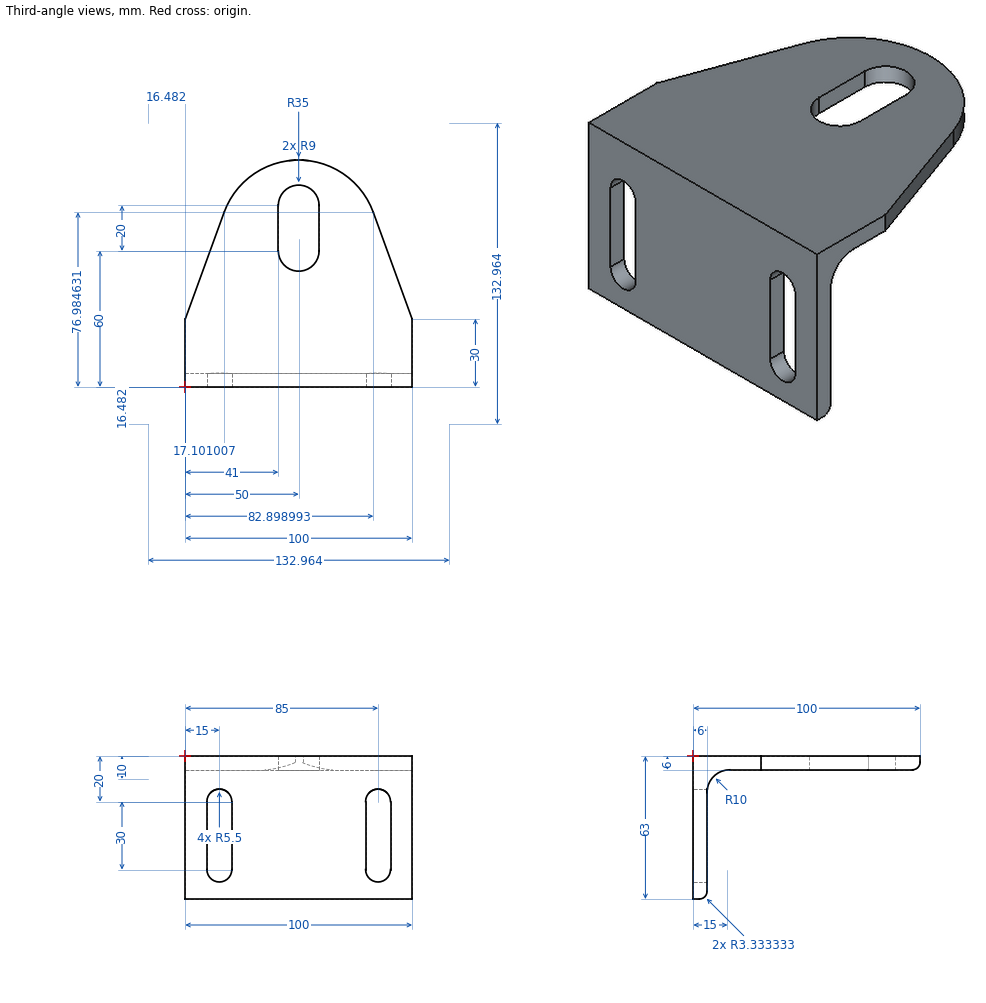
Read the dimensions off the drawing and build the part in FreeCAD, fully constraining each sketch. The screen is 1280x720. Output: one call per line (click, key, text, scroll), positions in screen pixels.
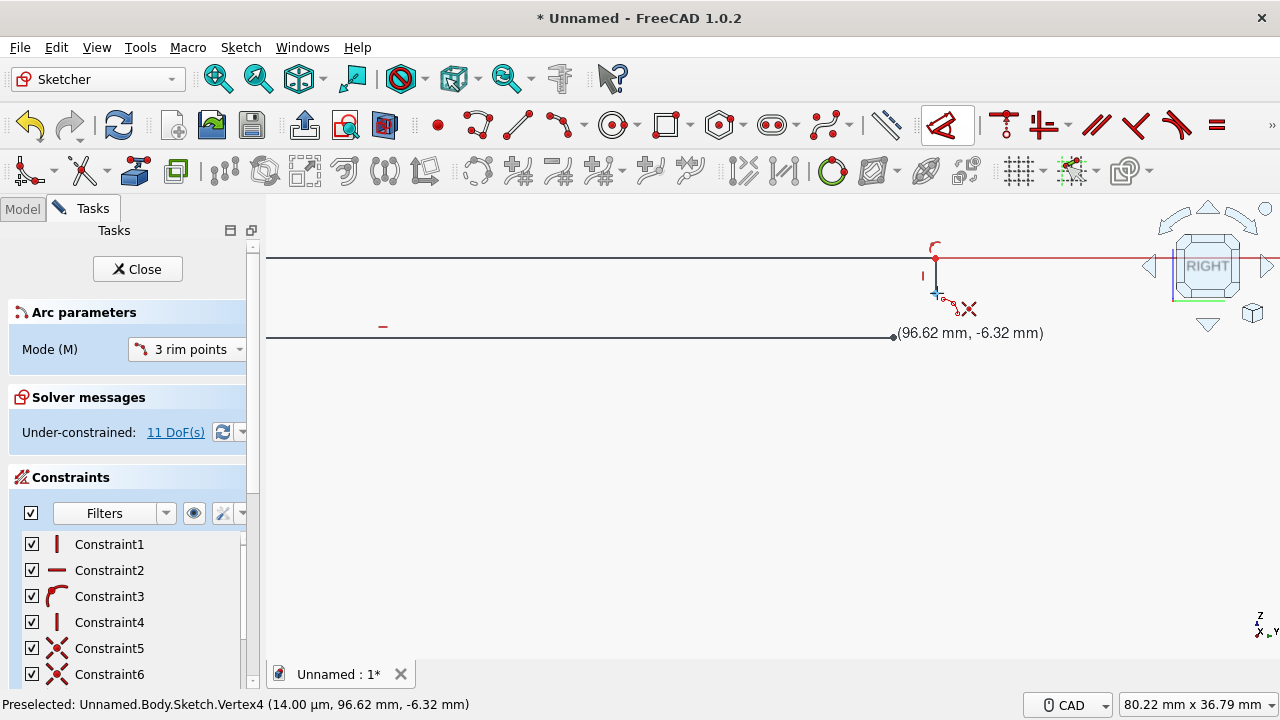
click(936, 294)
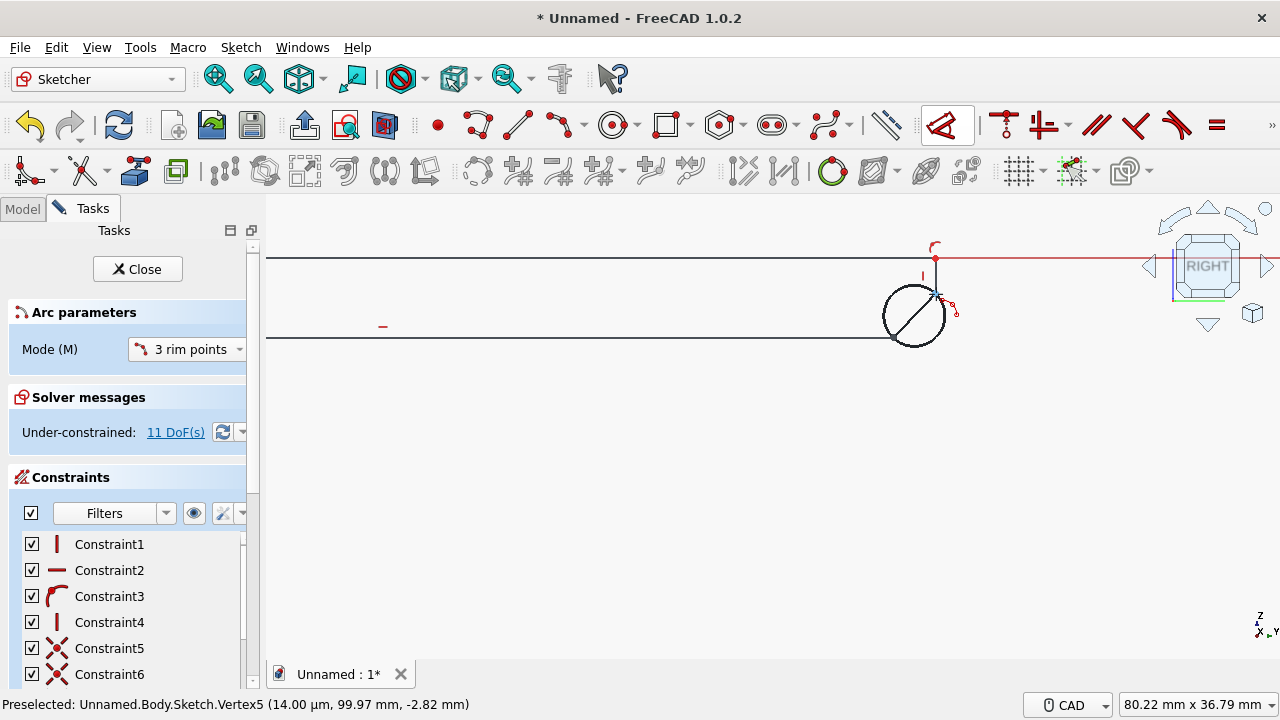
scroll(924, 322, up, 2)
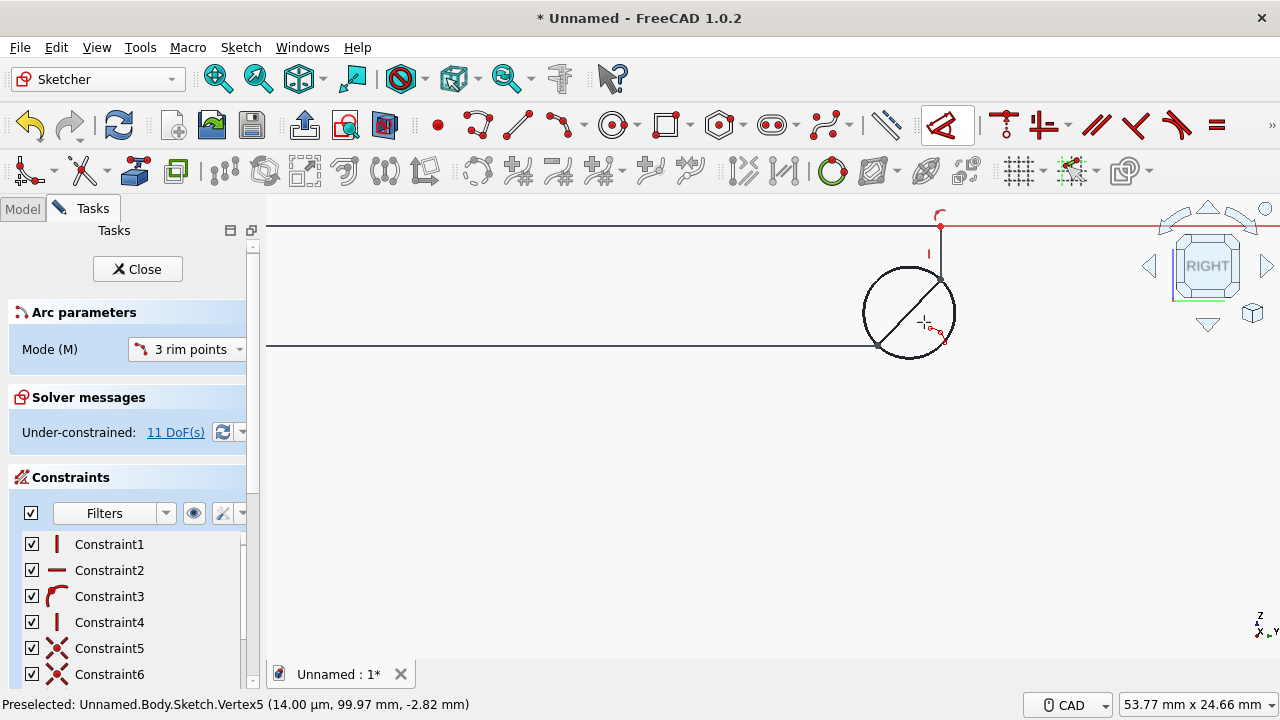
click(923, 321)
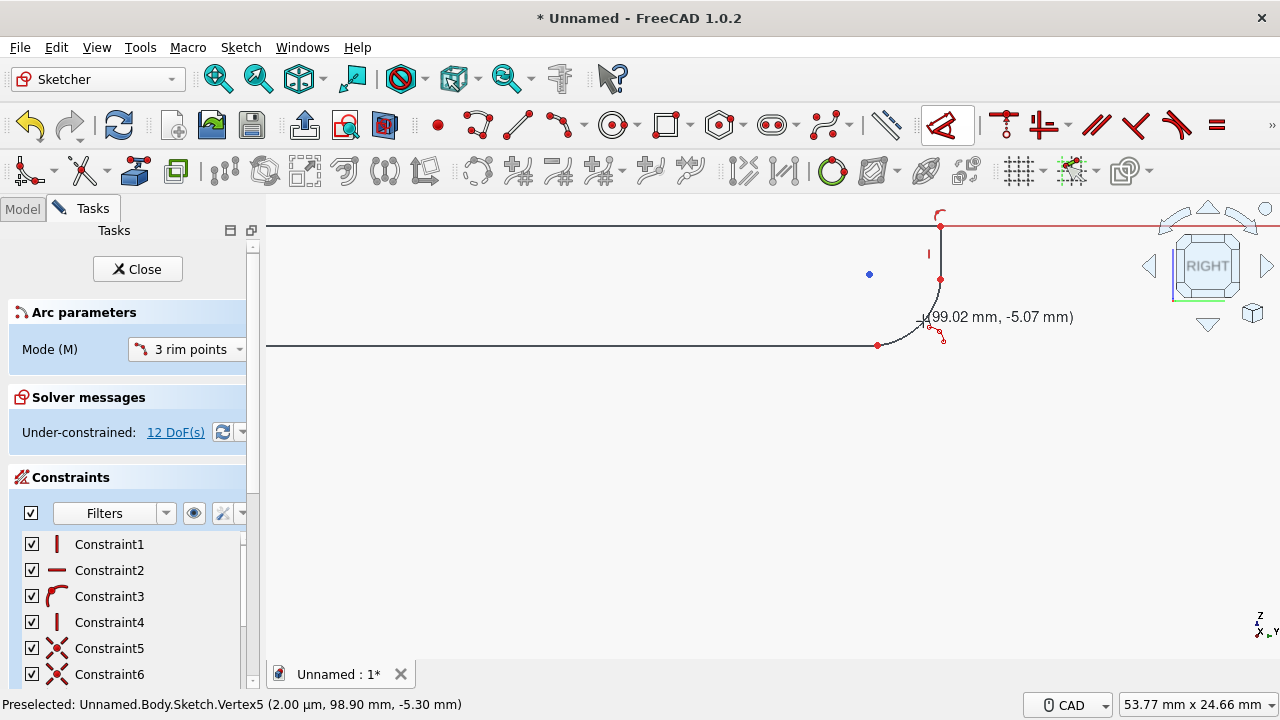
scroll(936, 298, down, 7)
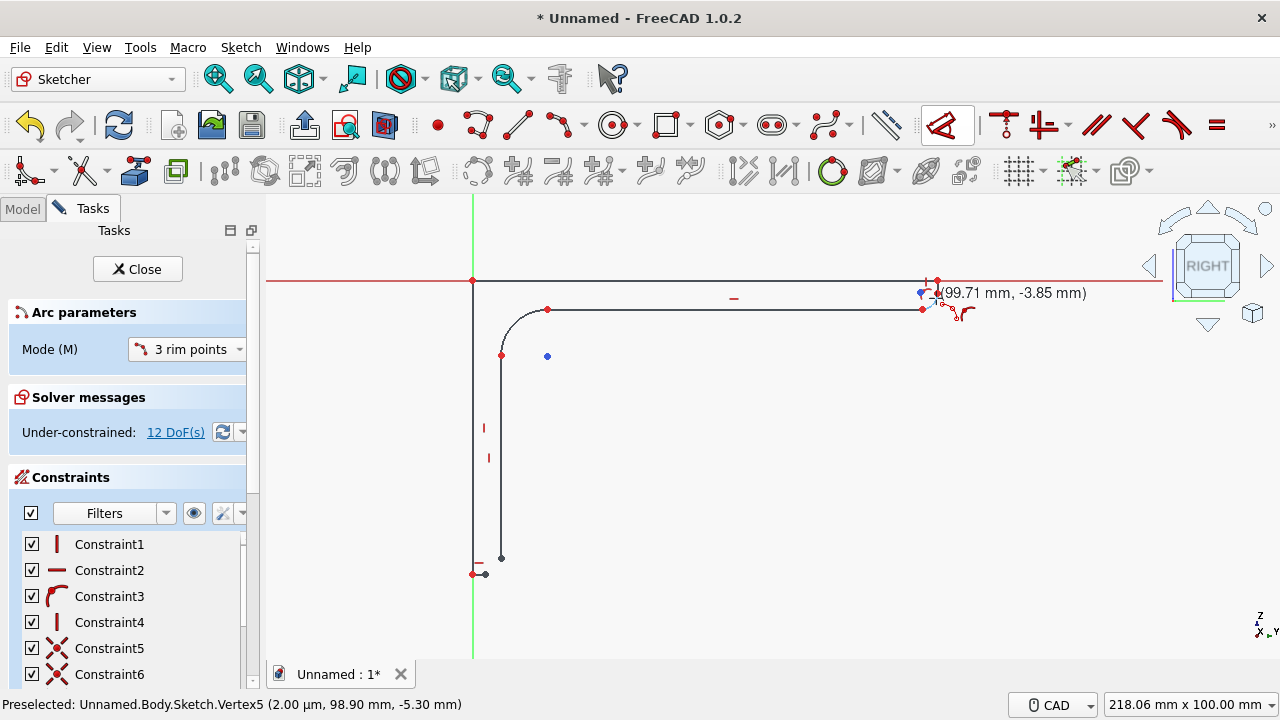
scroll(485, 573, up, 5)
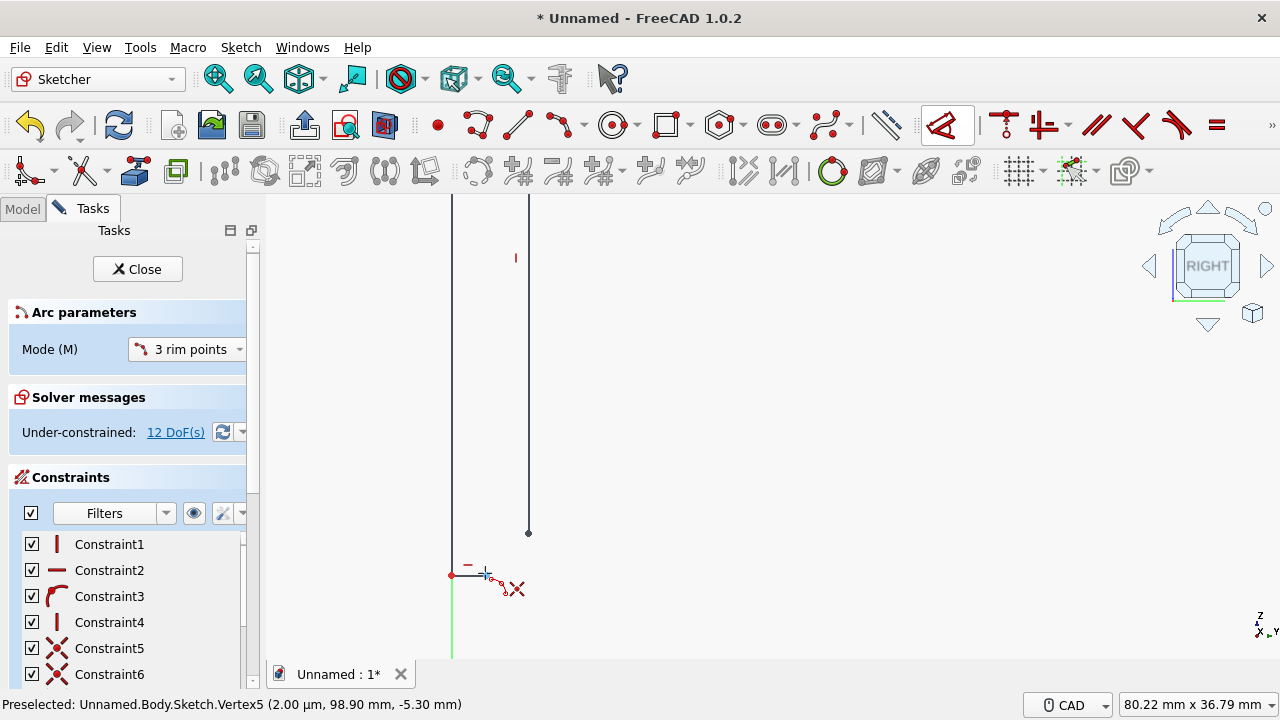
click(486, 576)
click(529, 533)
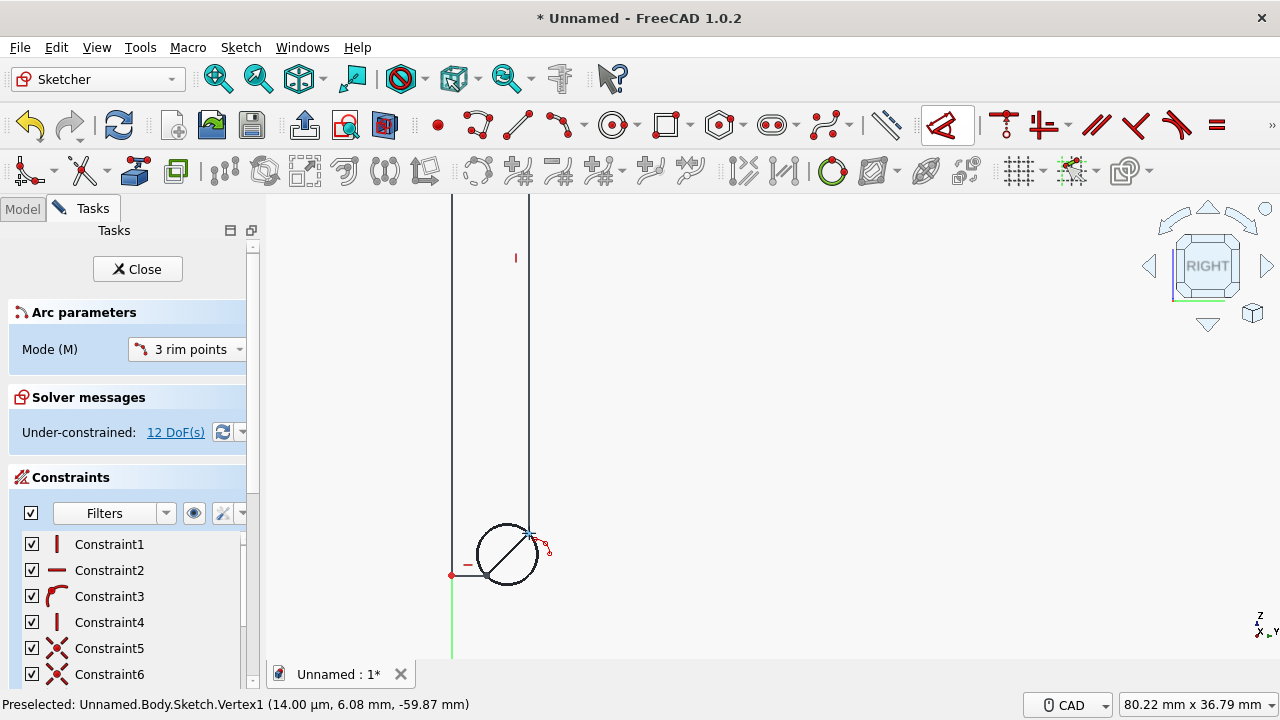
scroll(515, 561, up, 2)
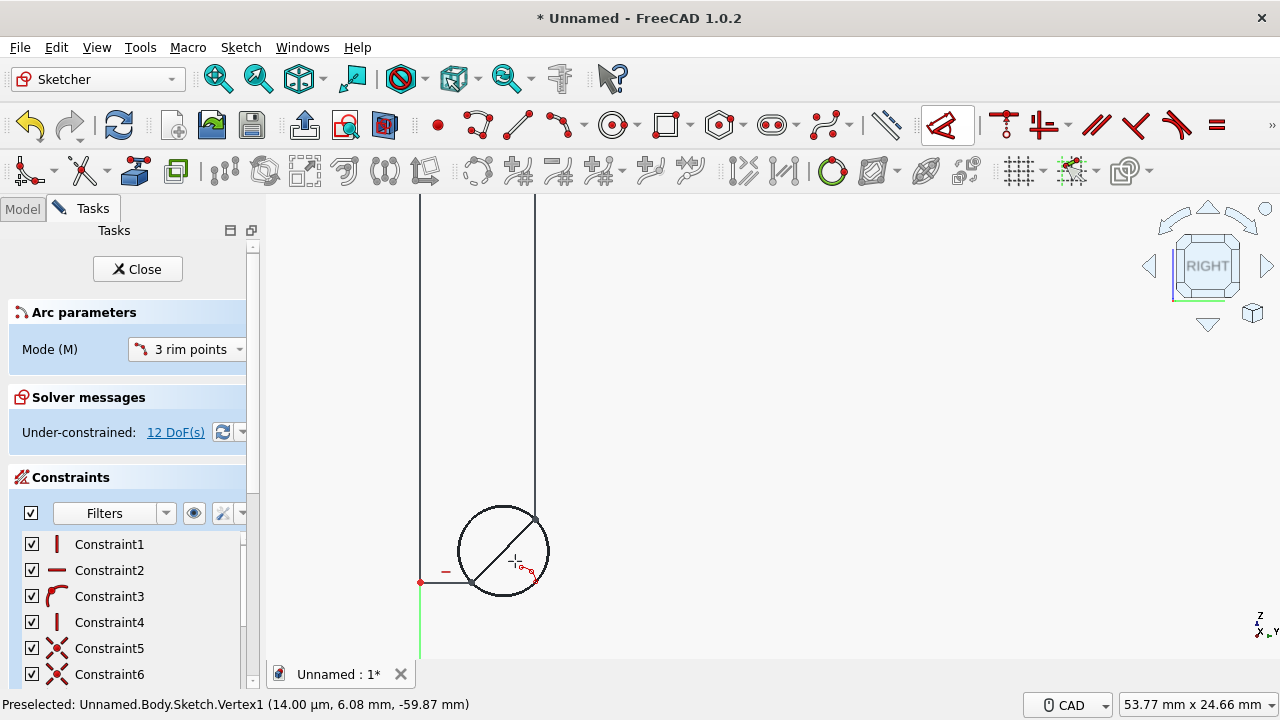
click(515, 560)
key(Escape)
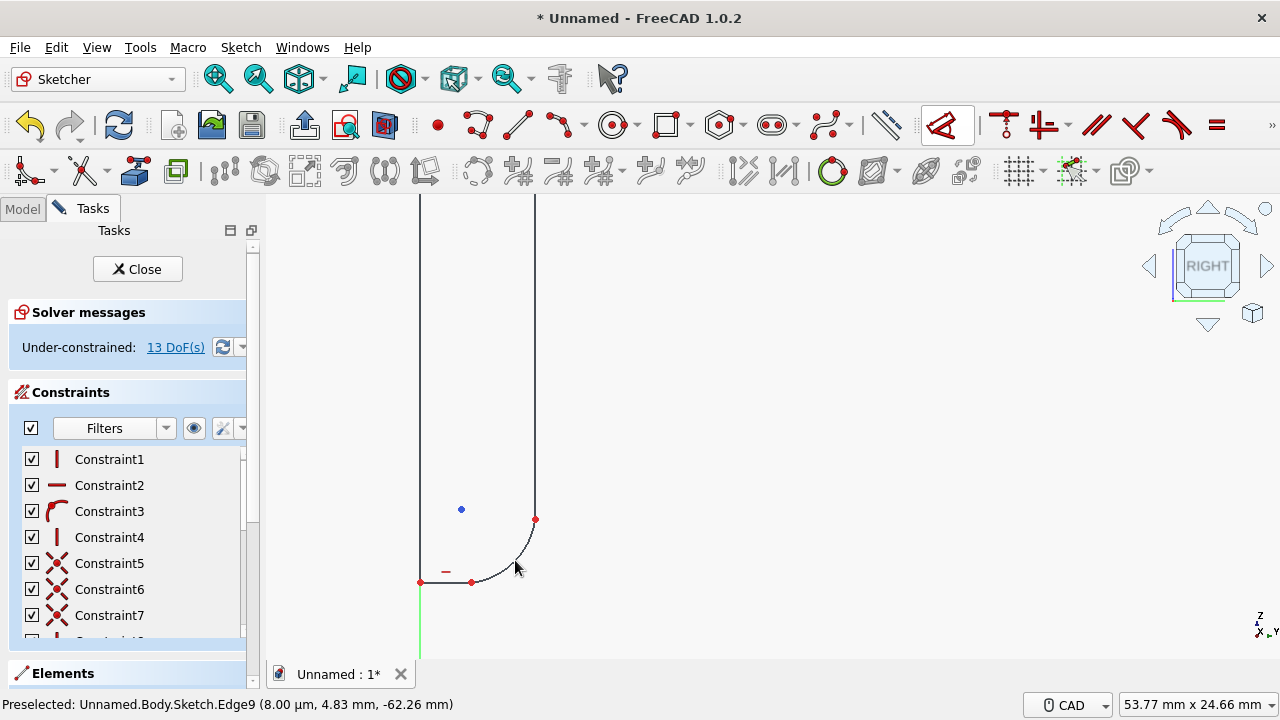
scroll(489, 571, down, 7)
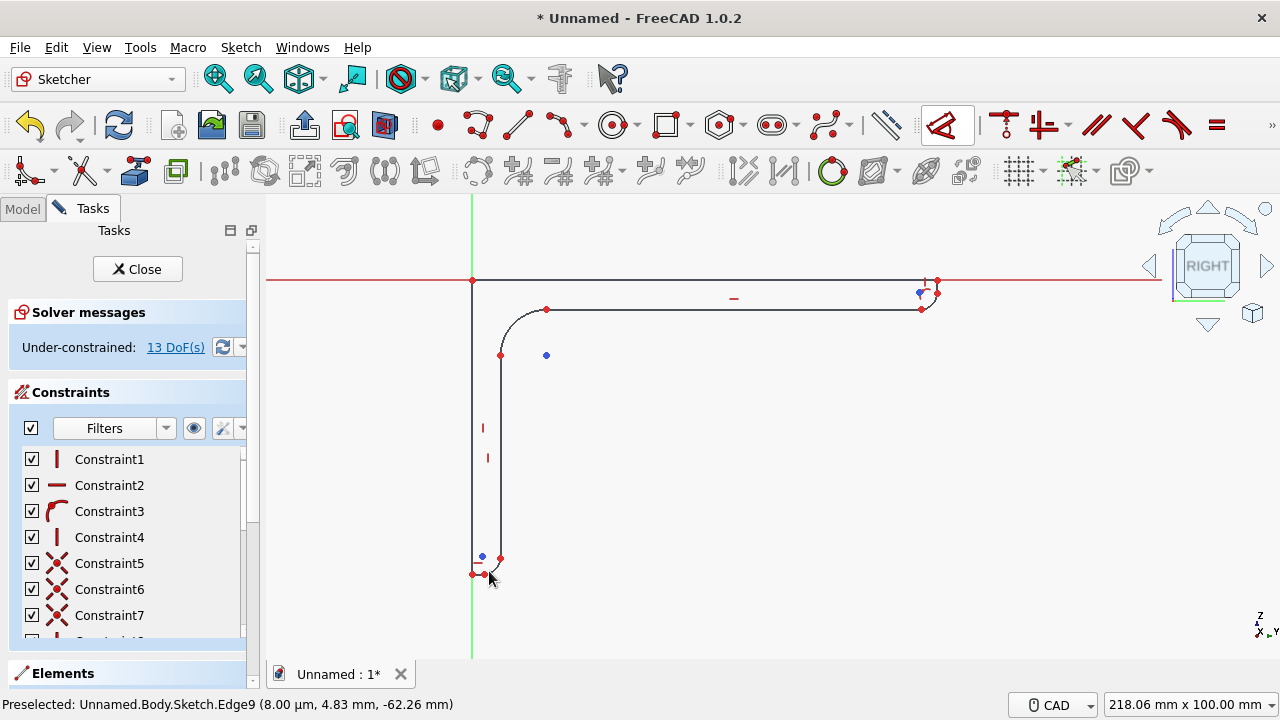
click(501, 498)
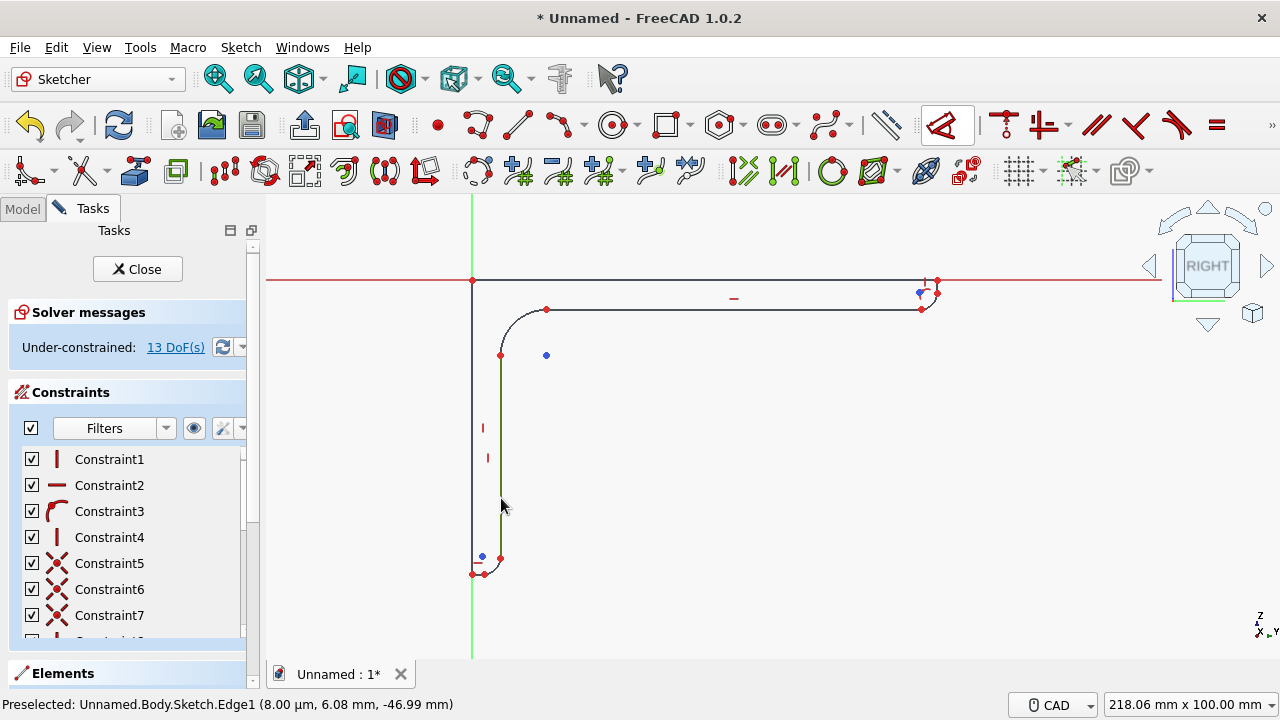
click(526, 315)